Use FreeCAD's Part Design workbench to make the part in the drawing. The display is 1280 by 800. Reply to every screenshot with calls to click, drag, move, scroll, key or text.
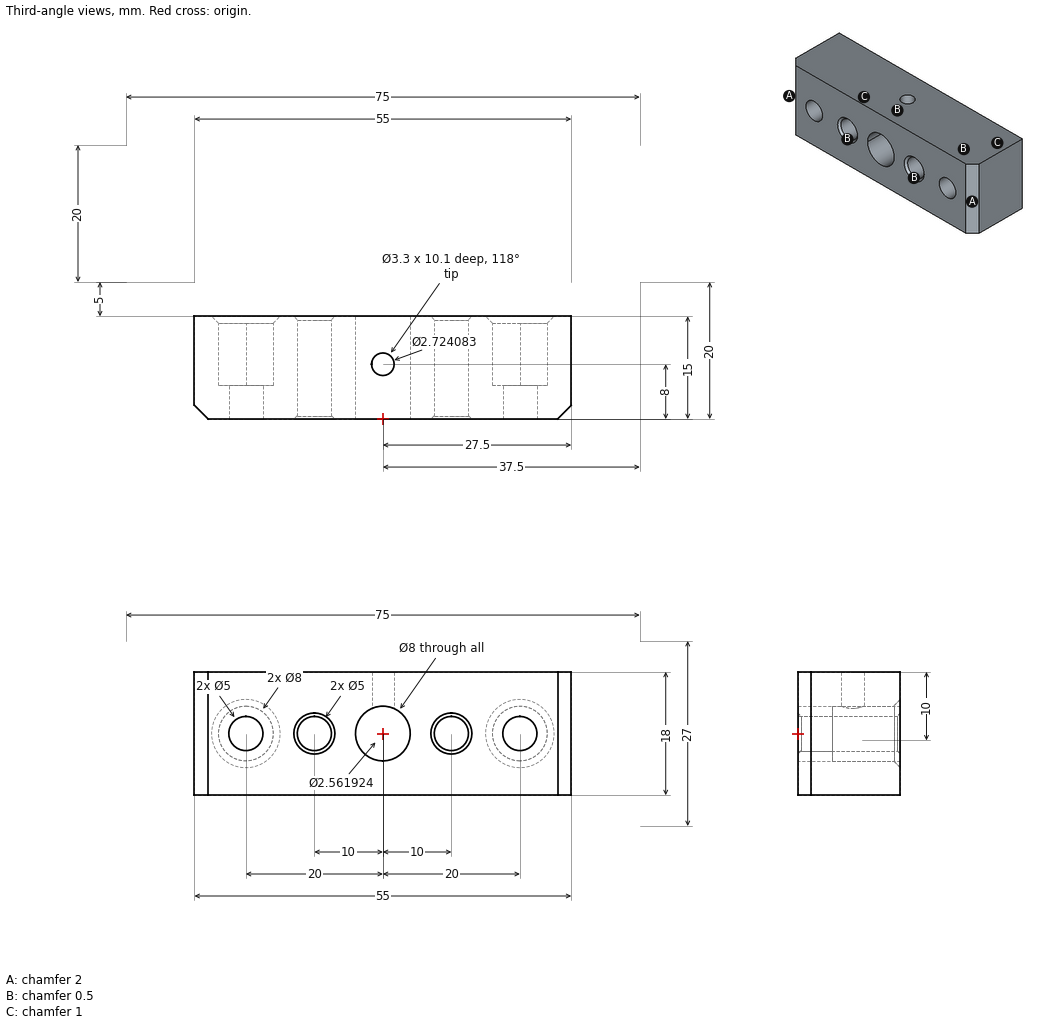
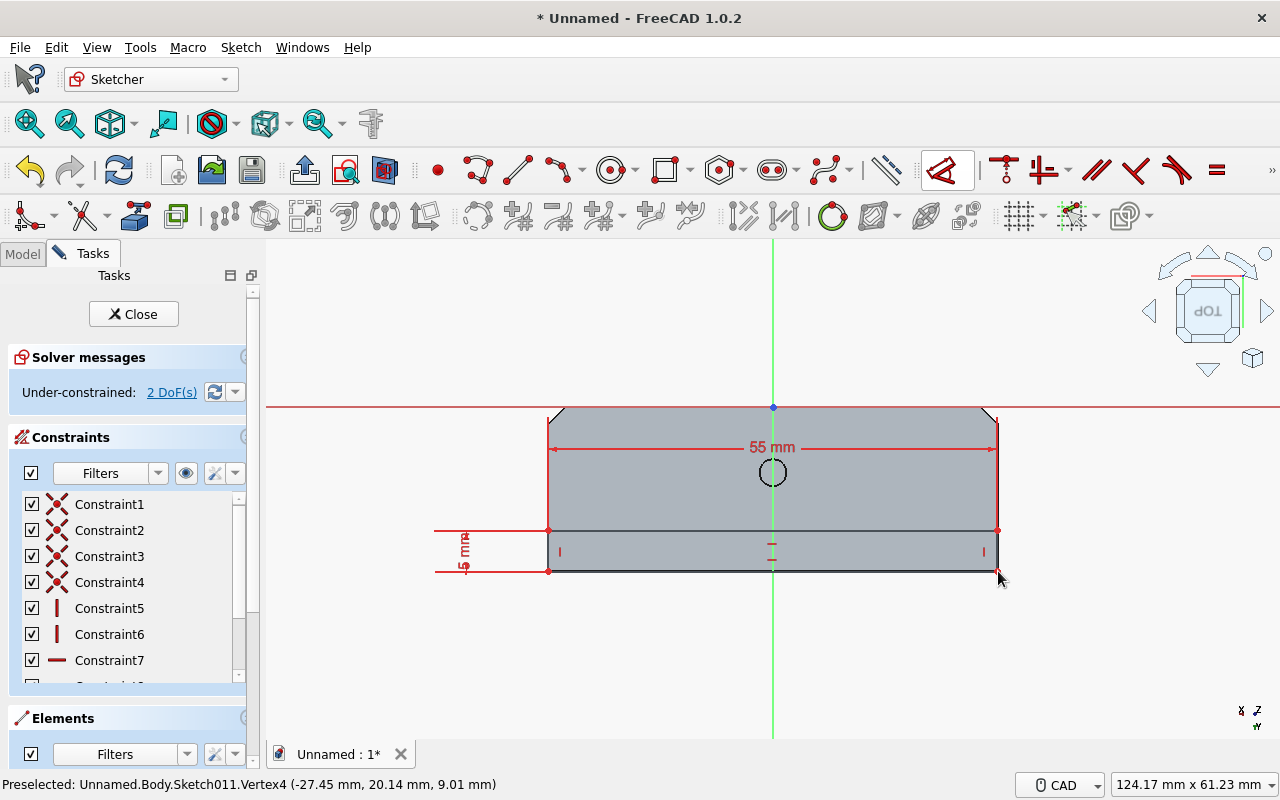
click(548, 531)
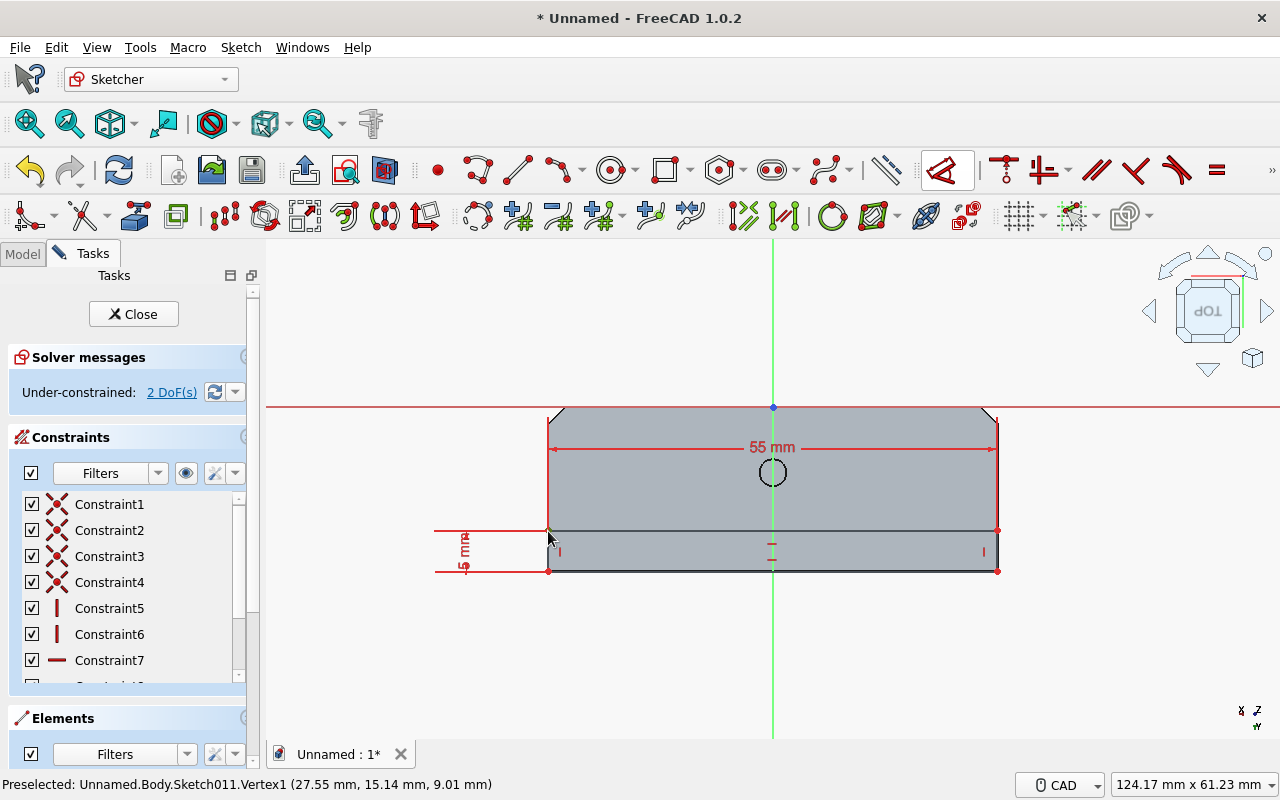
click(968, 170)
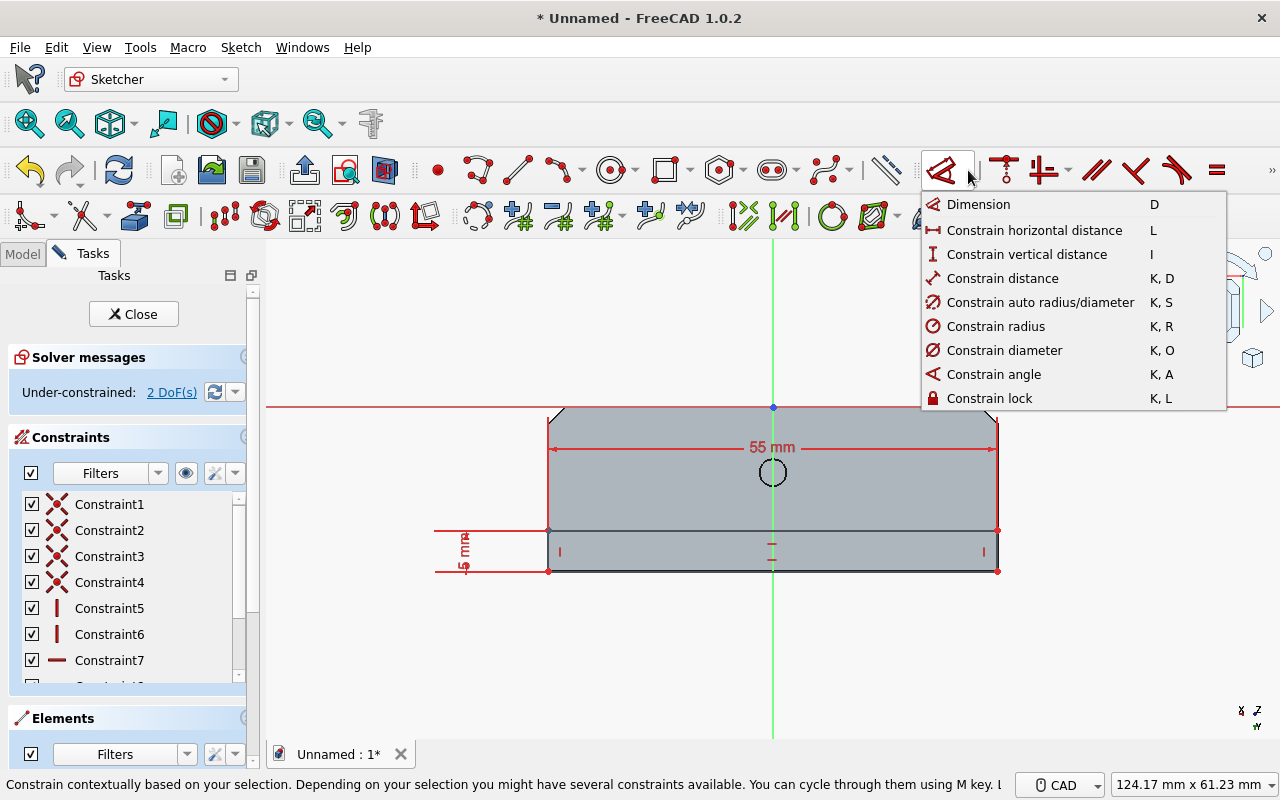
click(1074, 254)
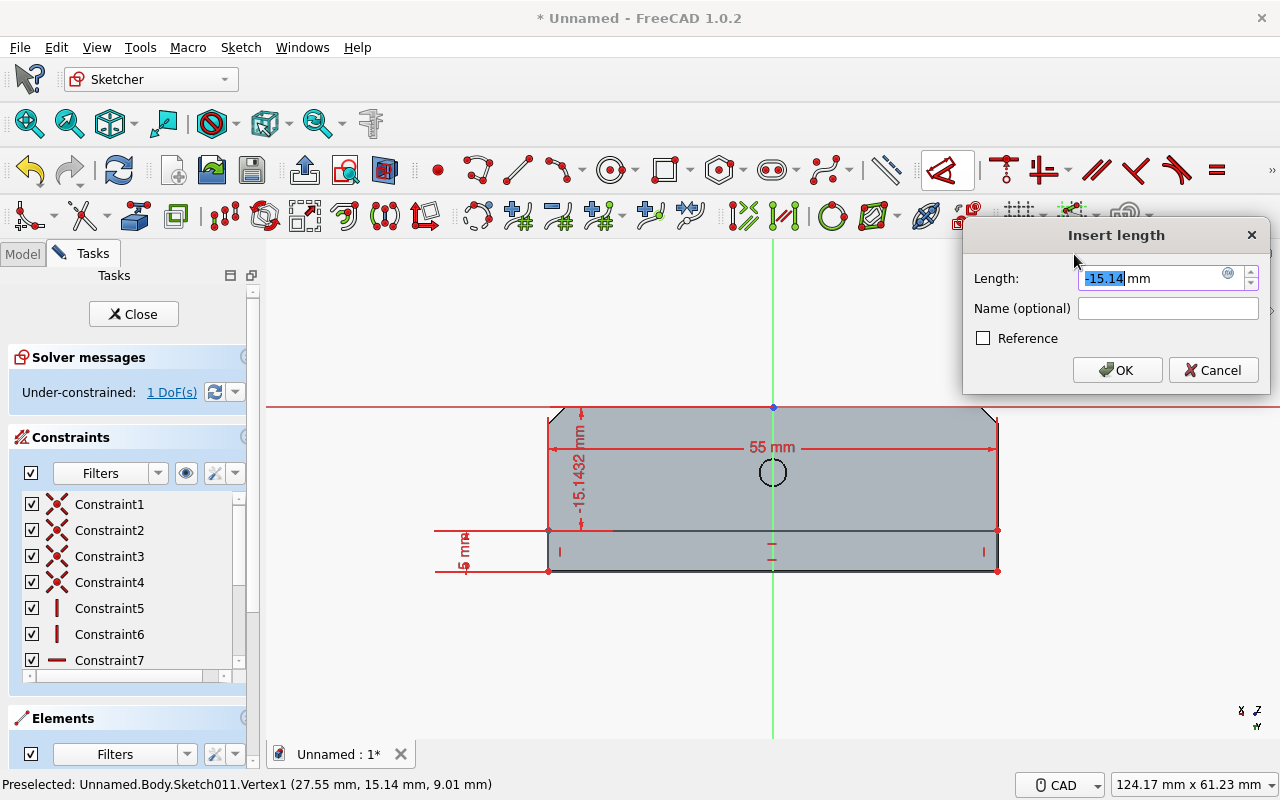
text(-15)
key(Return)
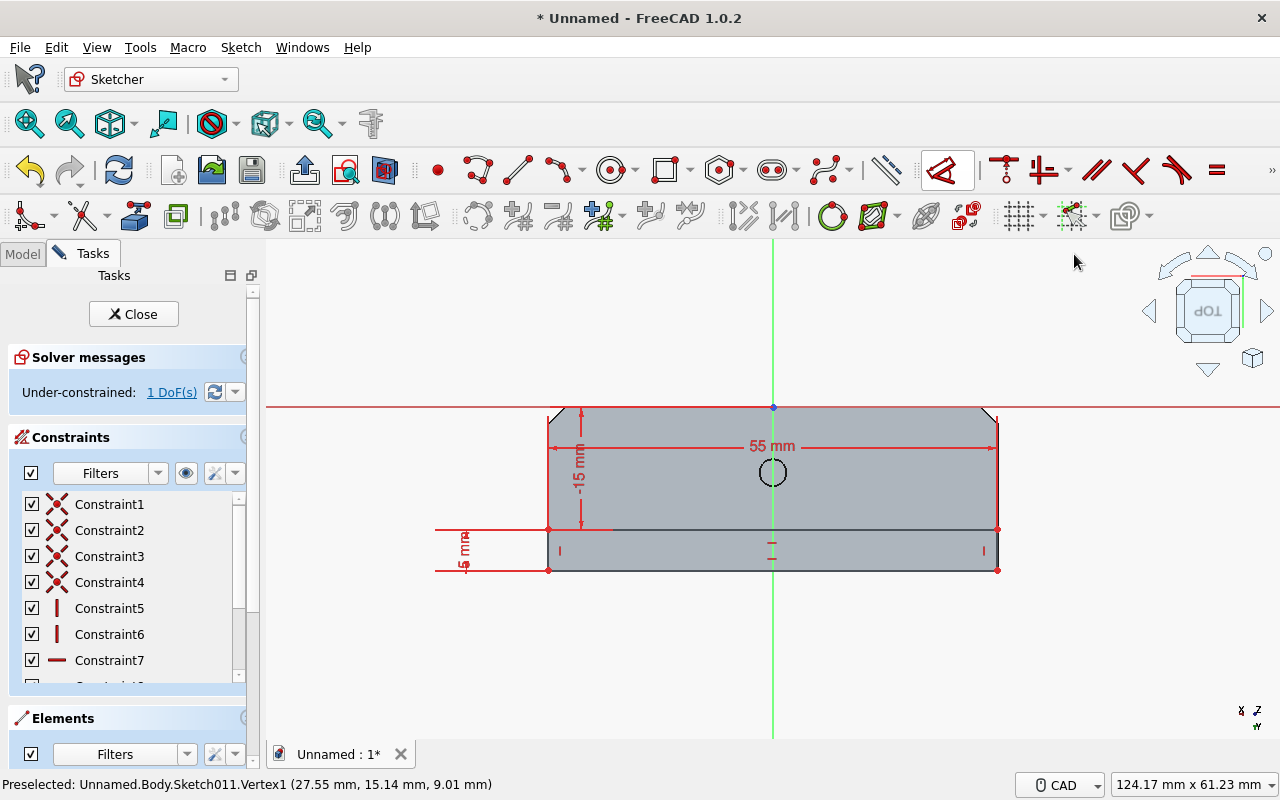
click(548, 530)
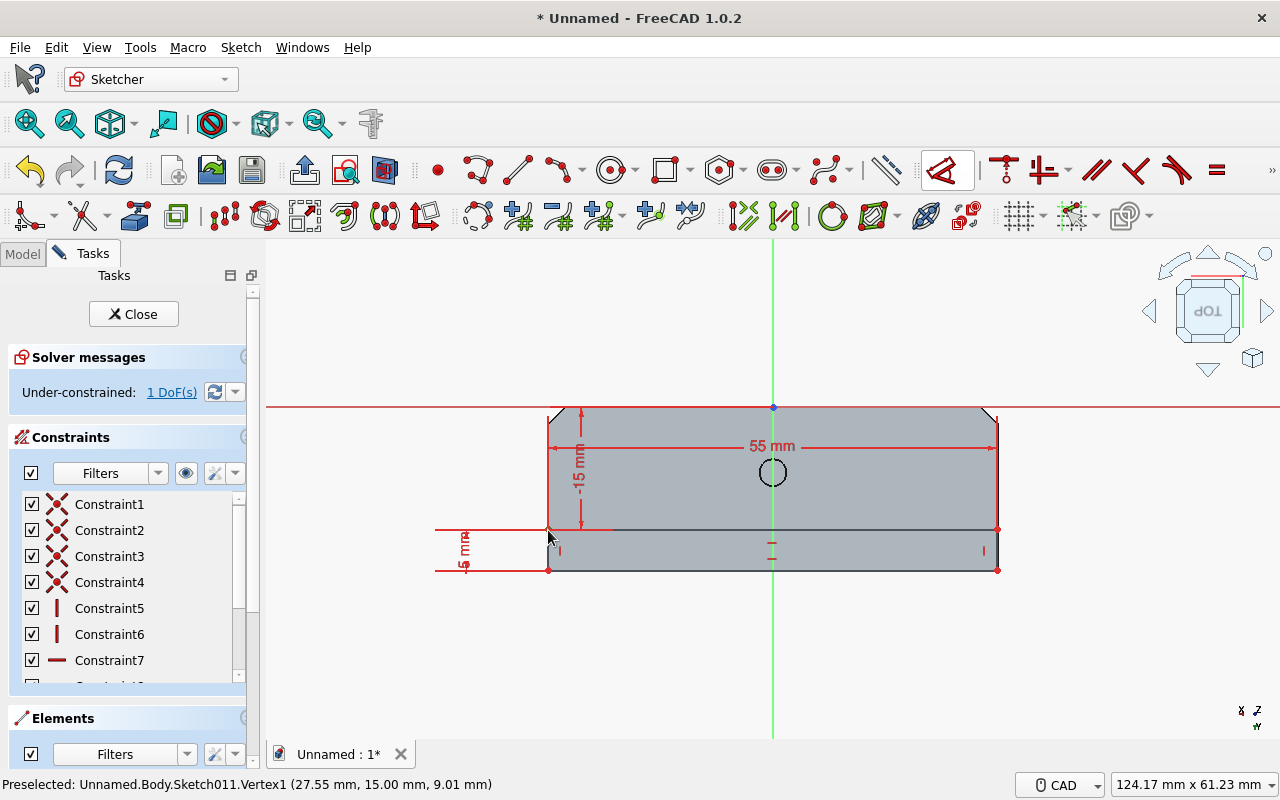
key(l)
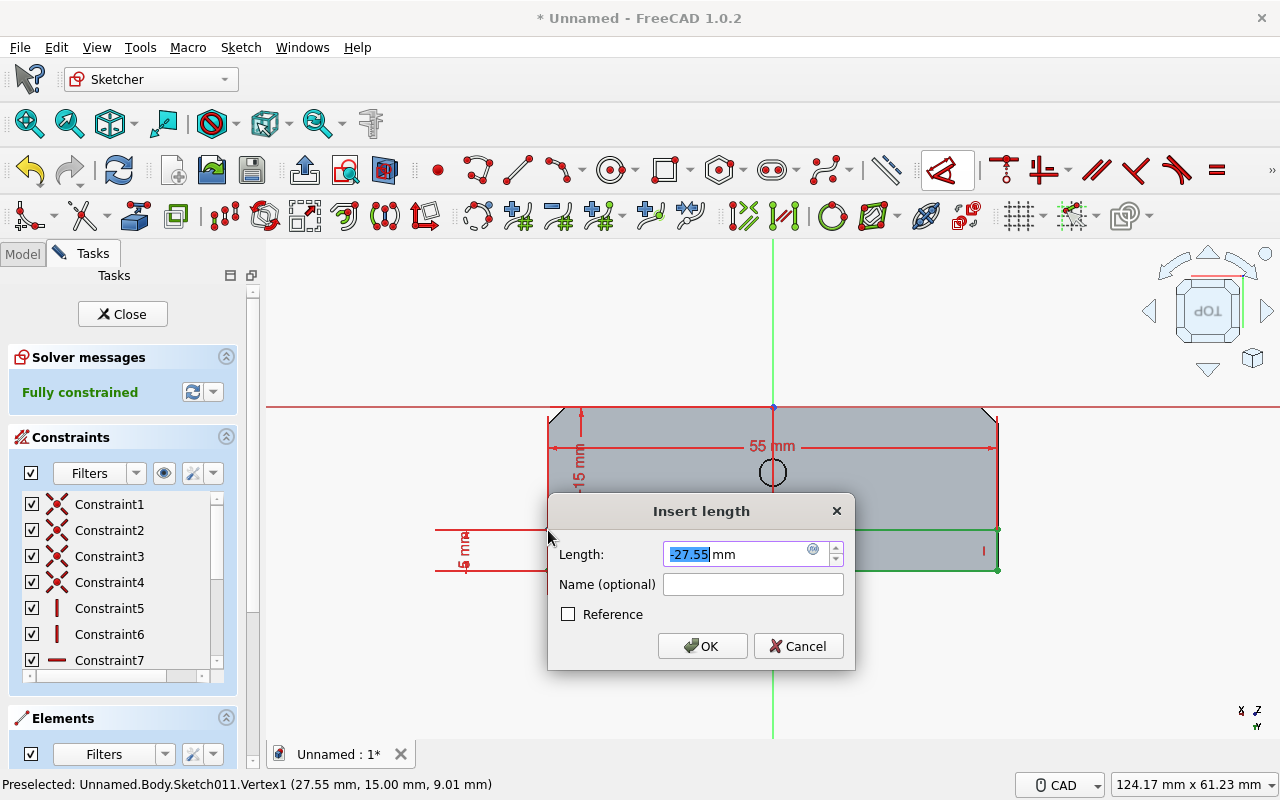
text(-27.5)
key(Return)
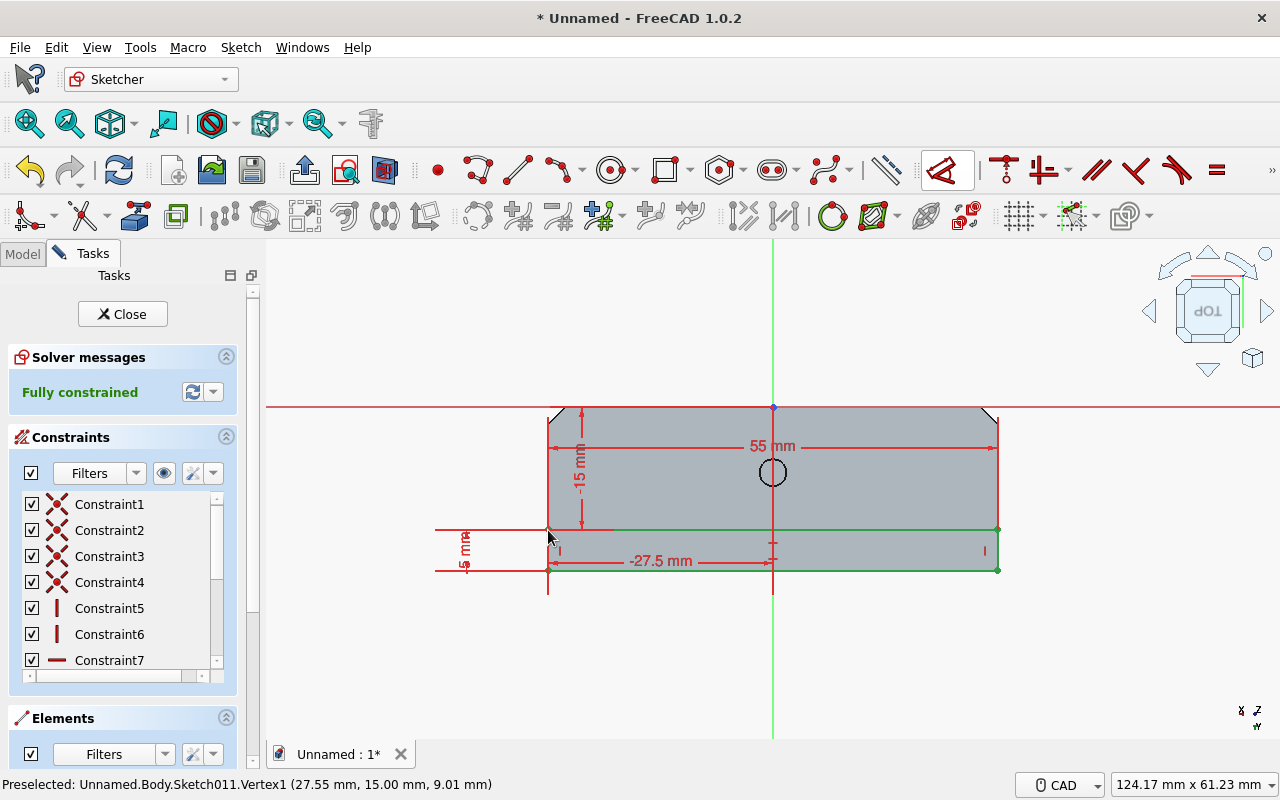
click(123, 314)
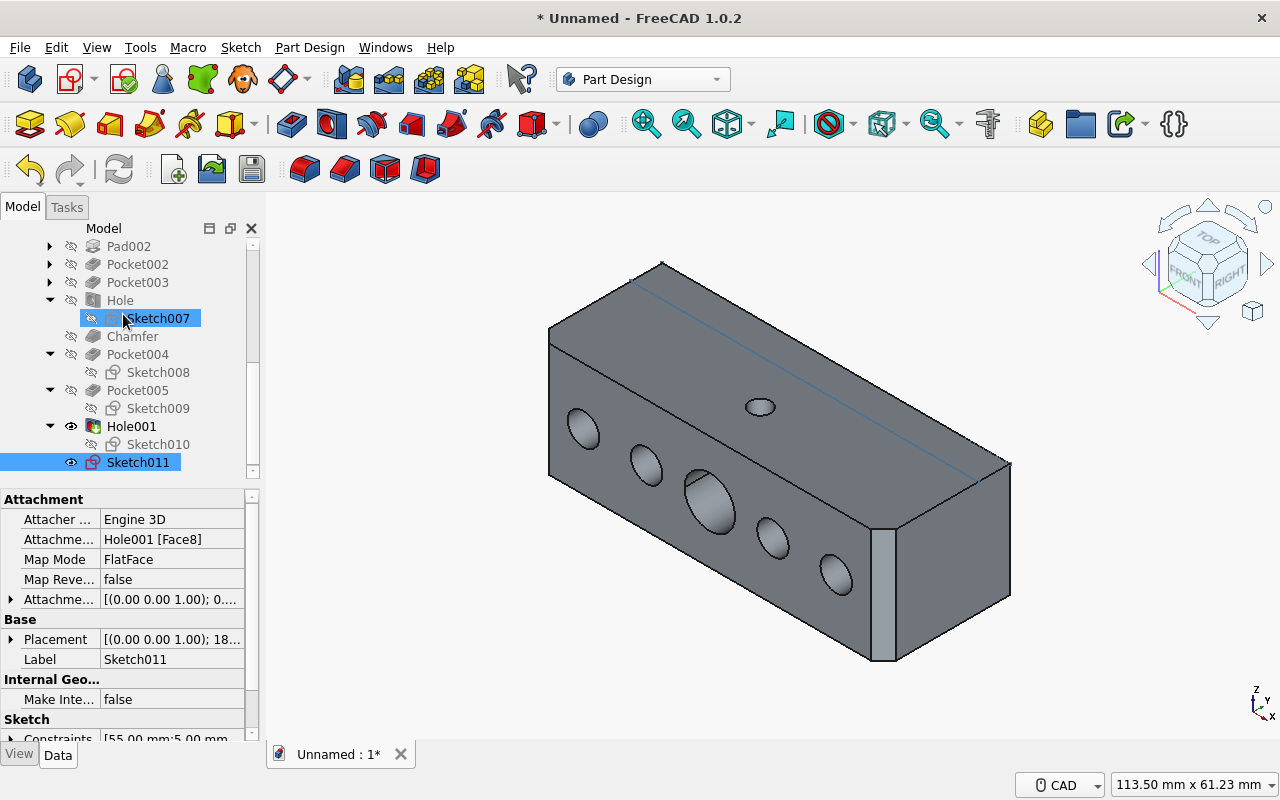
click(292, 124)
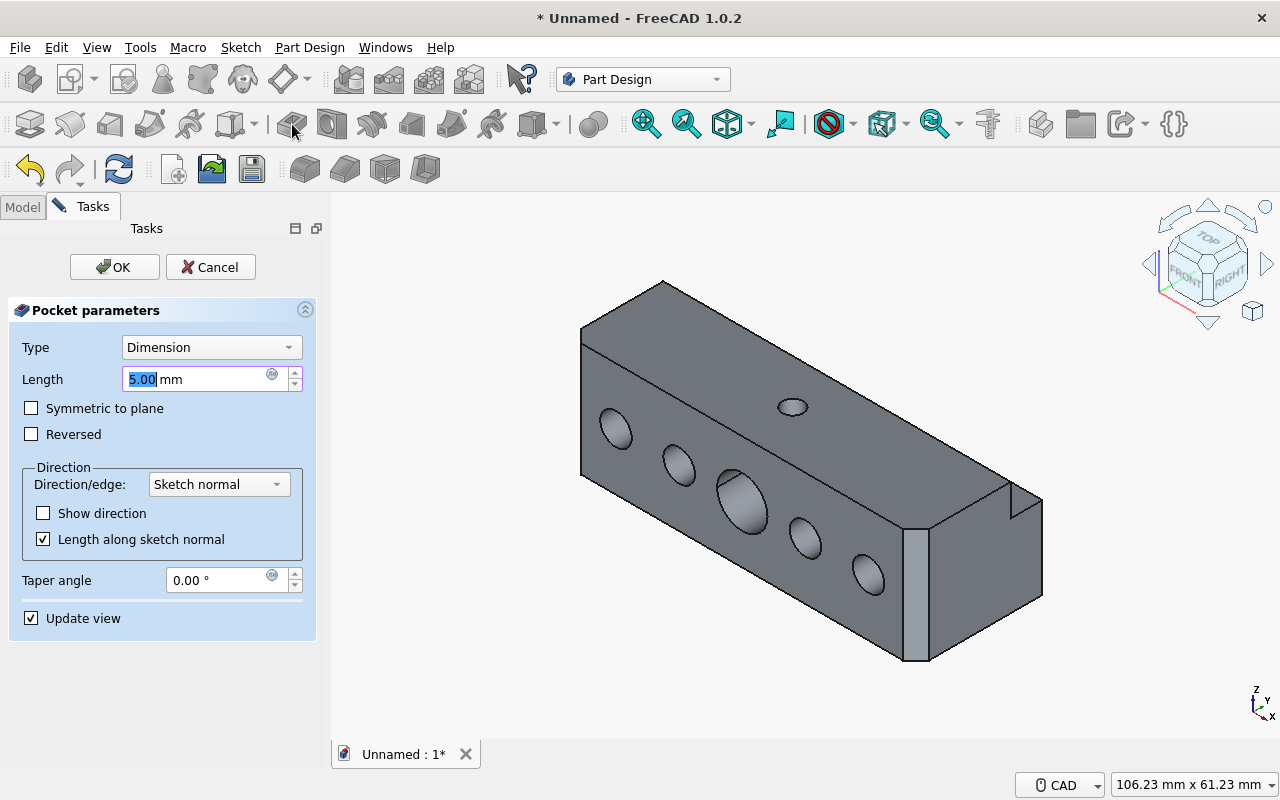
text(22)
key(Tab)